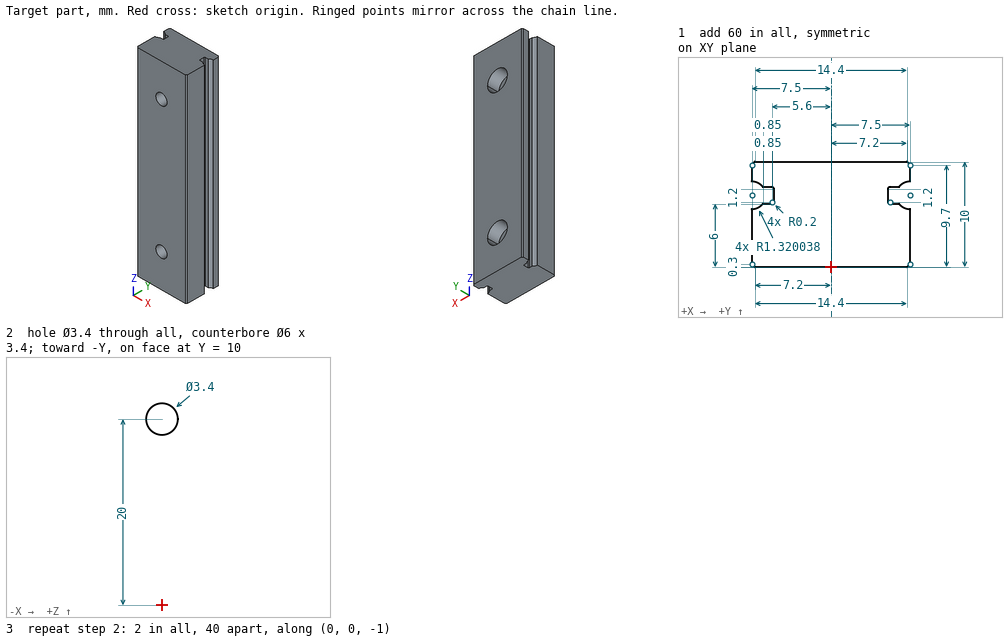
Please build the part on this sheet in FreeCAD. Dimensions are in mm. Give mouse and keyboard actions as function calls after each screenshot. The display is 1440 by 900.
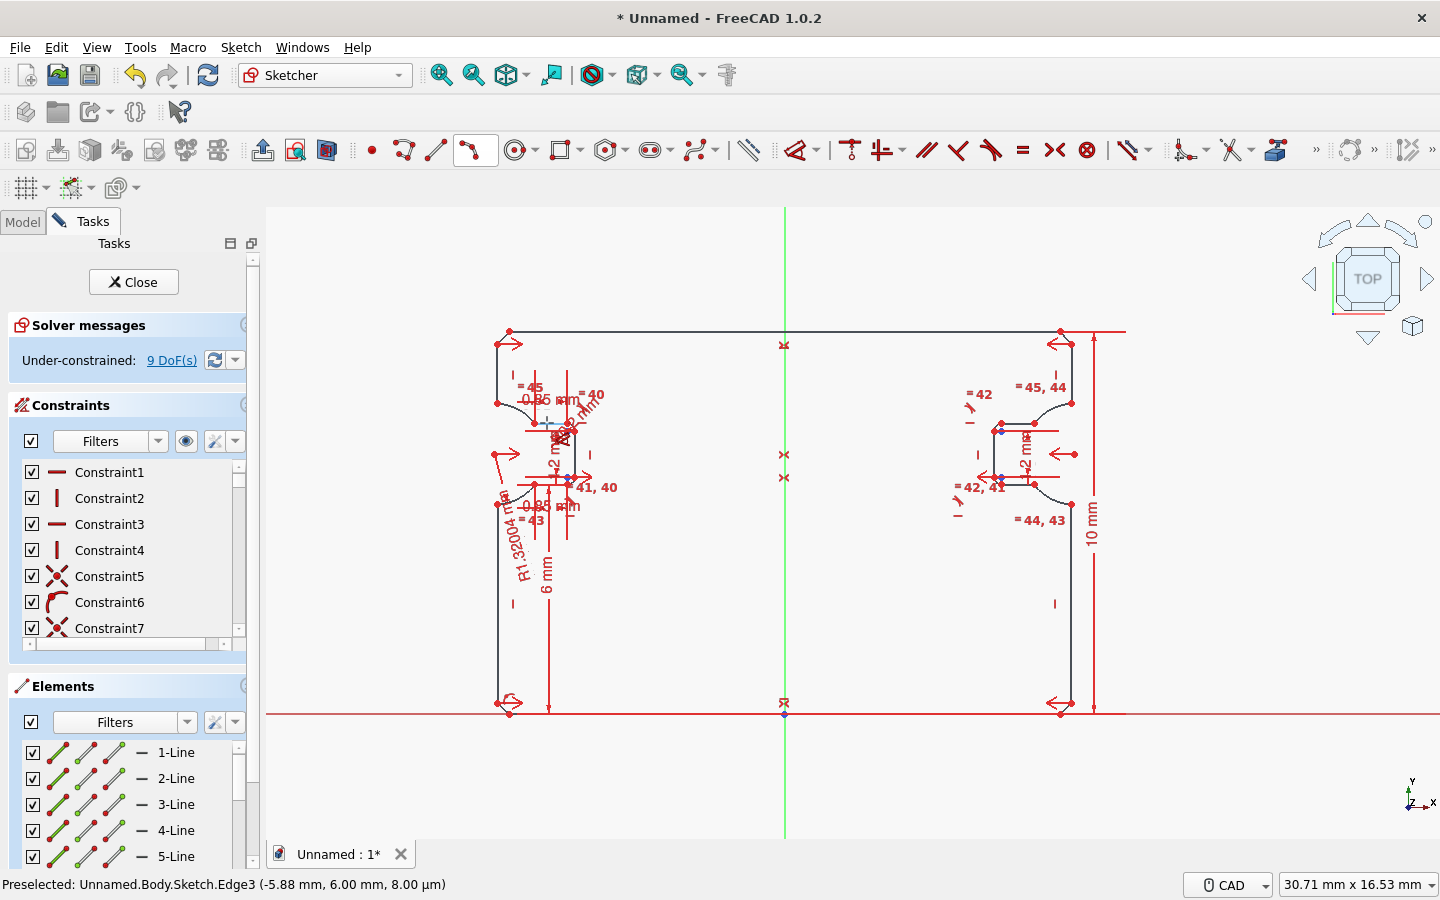
click(674, 714)
click(658, 748)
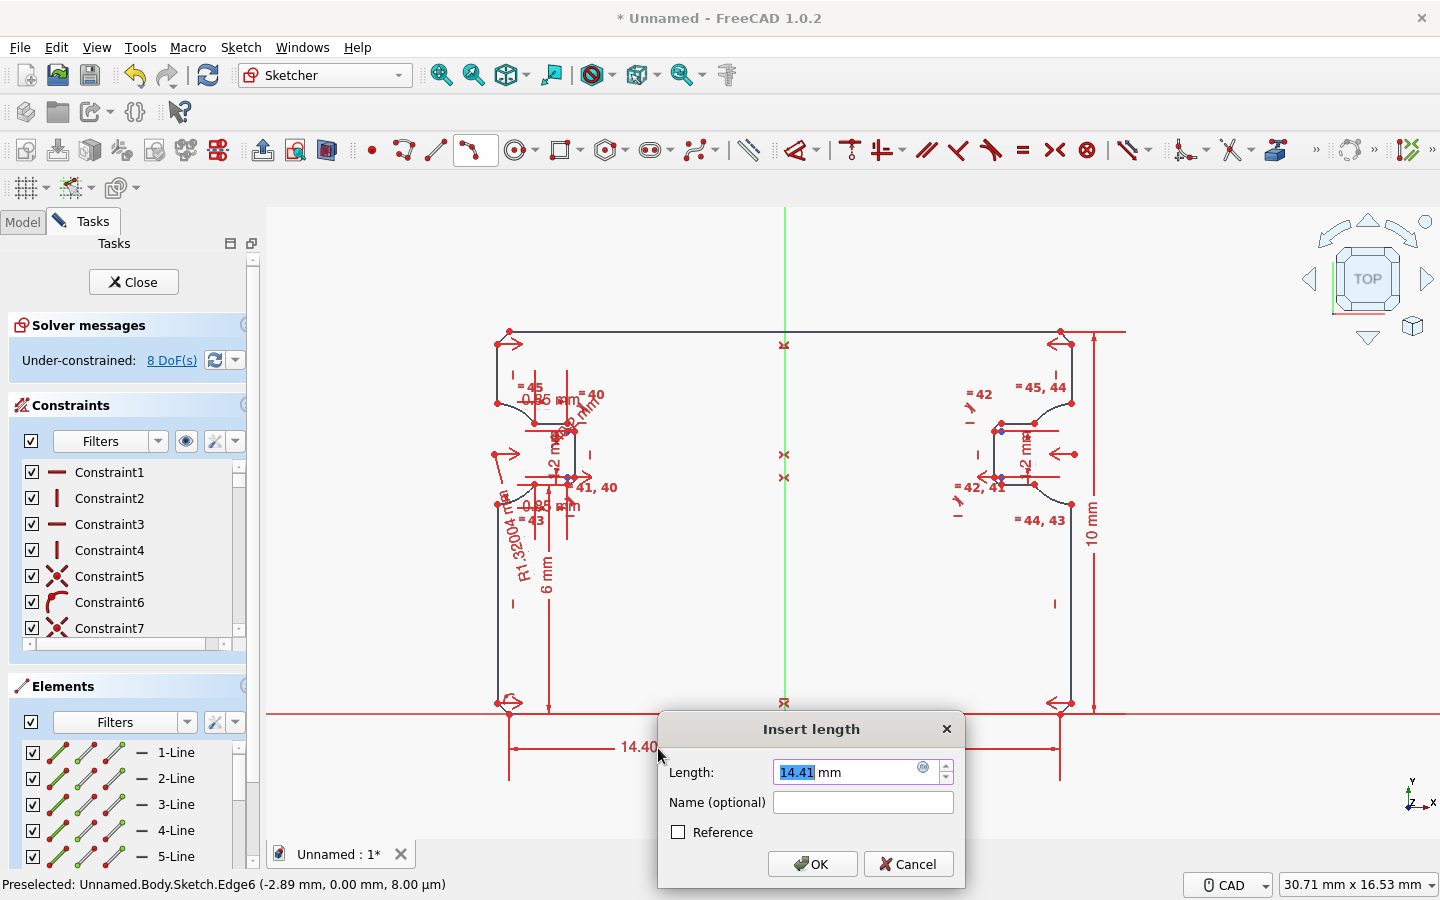
text(14.4)
key(Return)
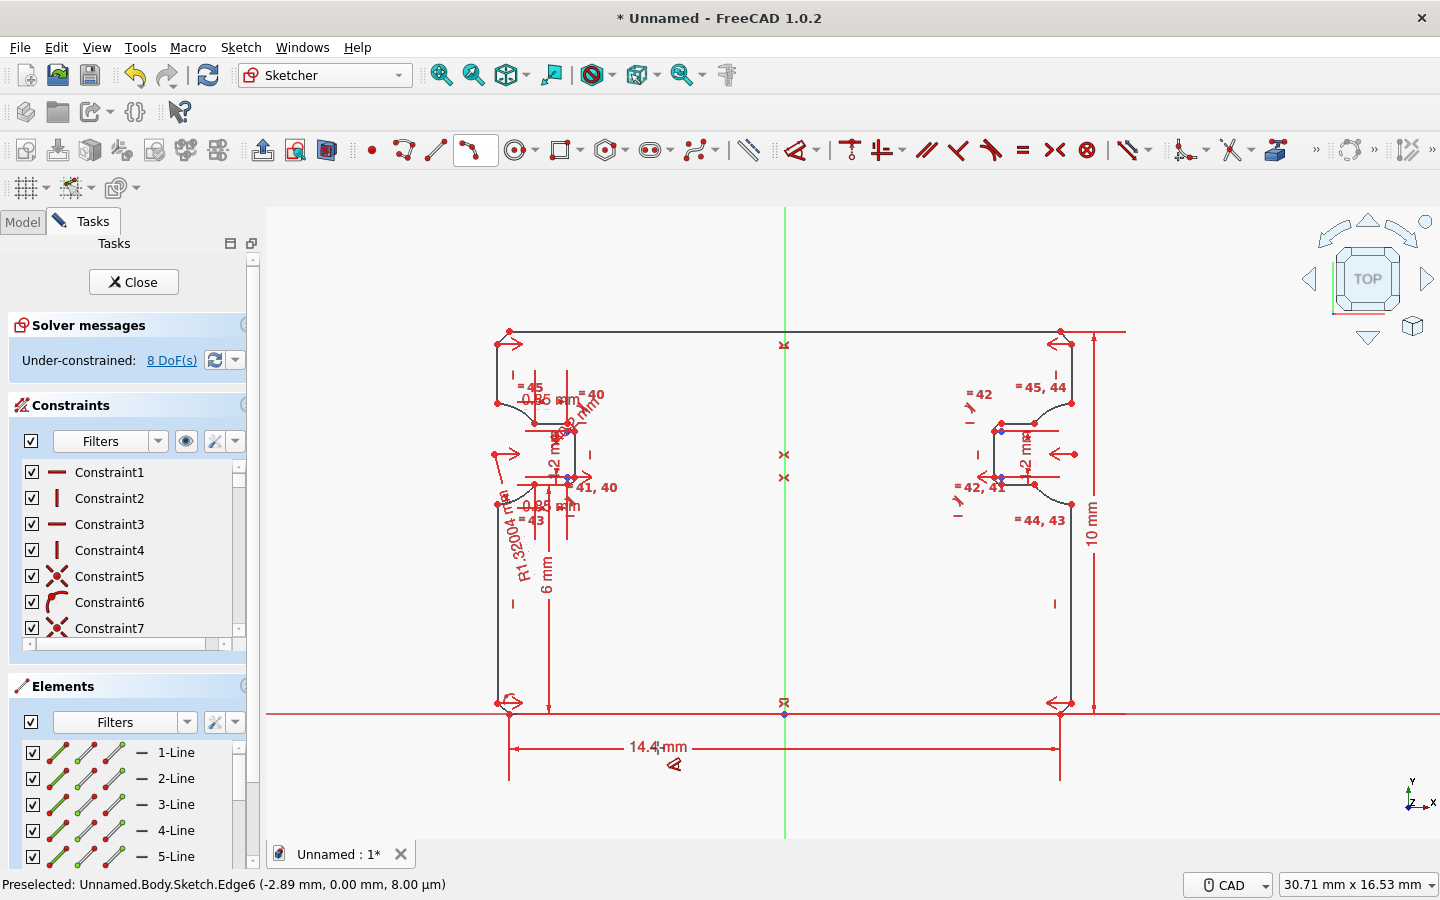
click(895, 332)
click(658, 298)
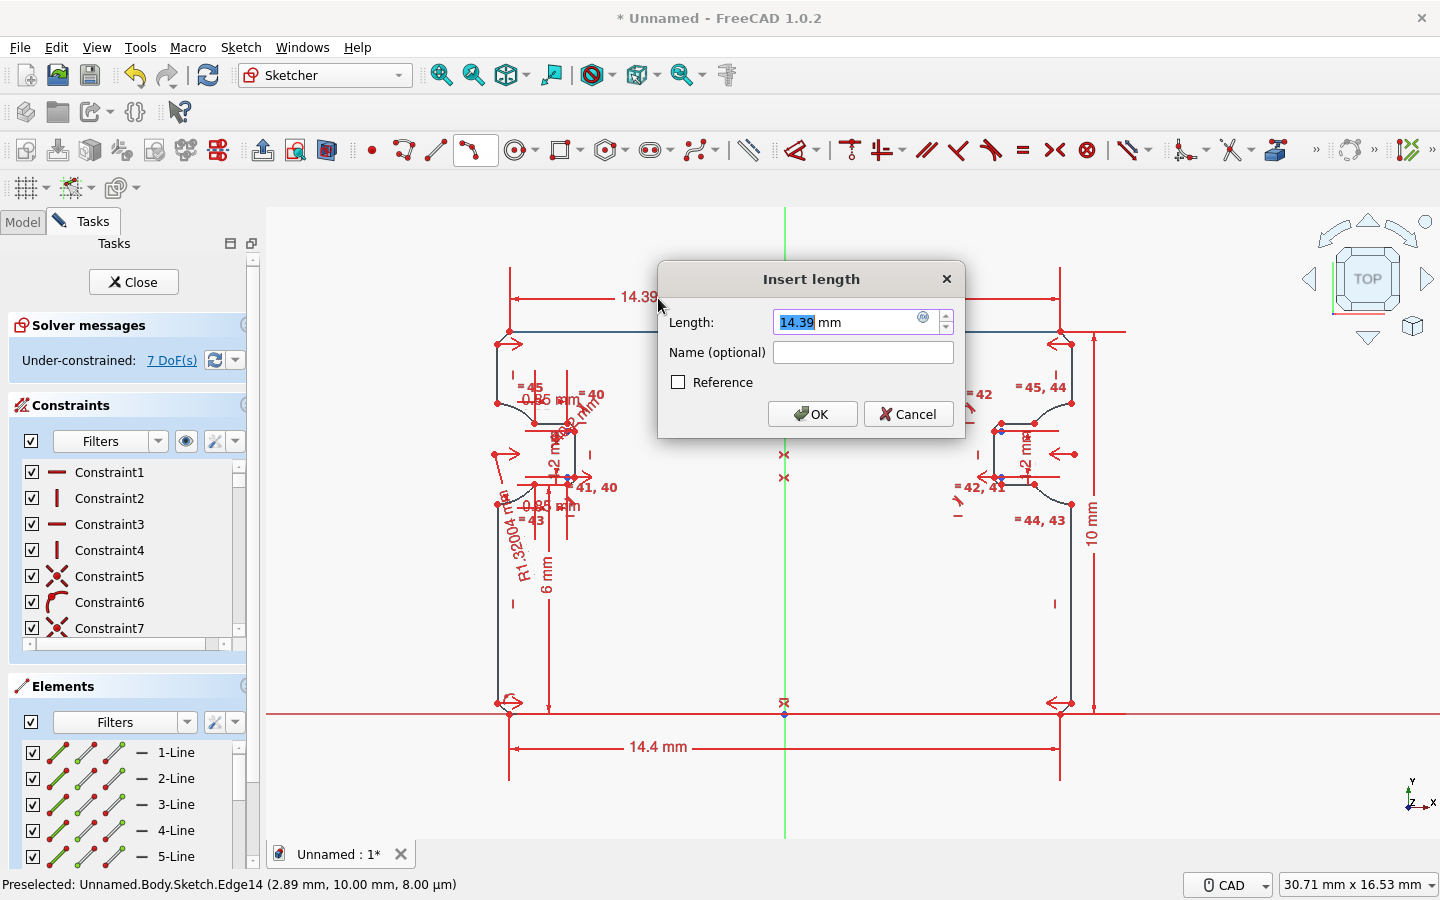
text(14.4)
key(Return)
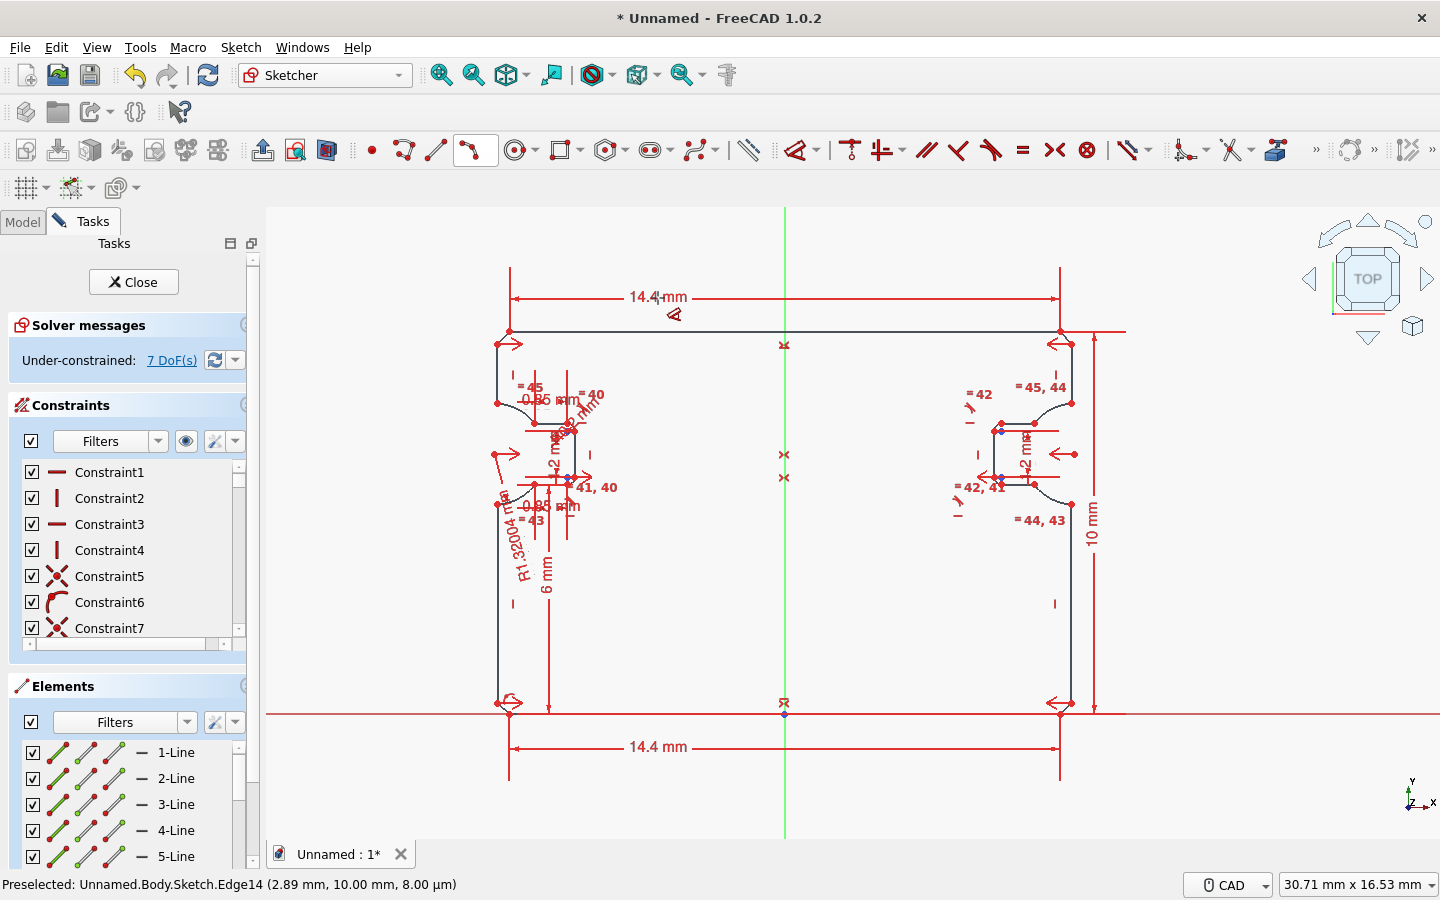
scroll(567, 424, up, 3)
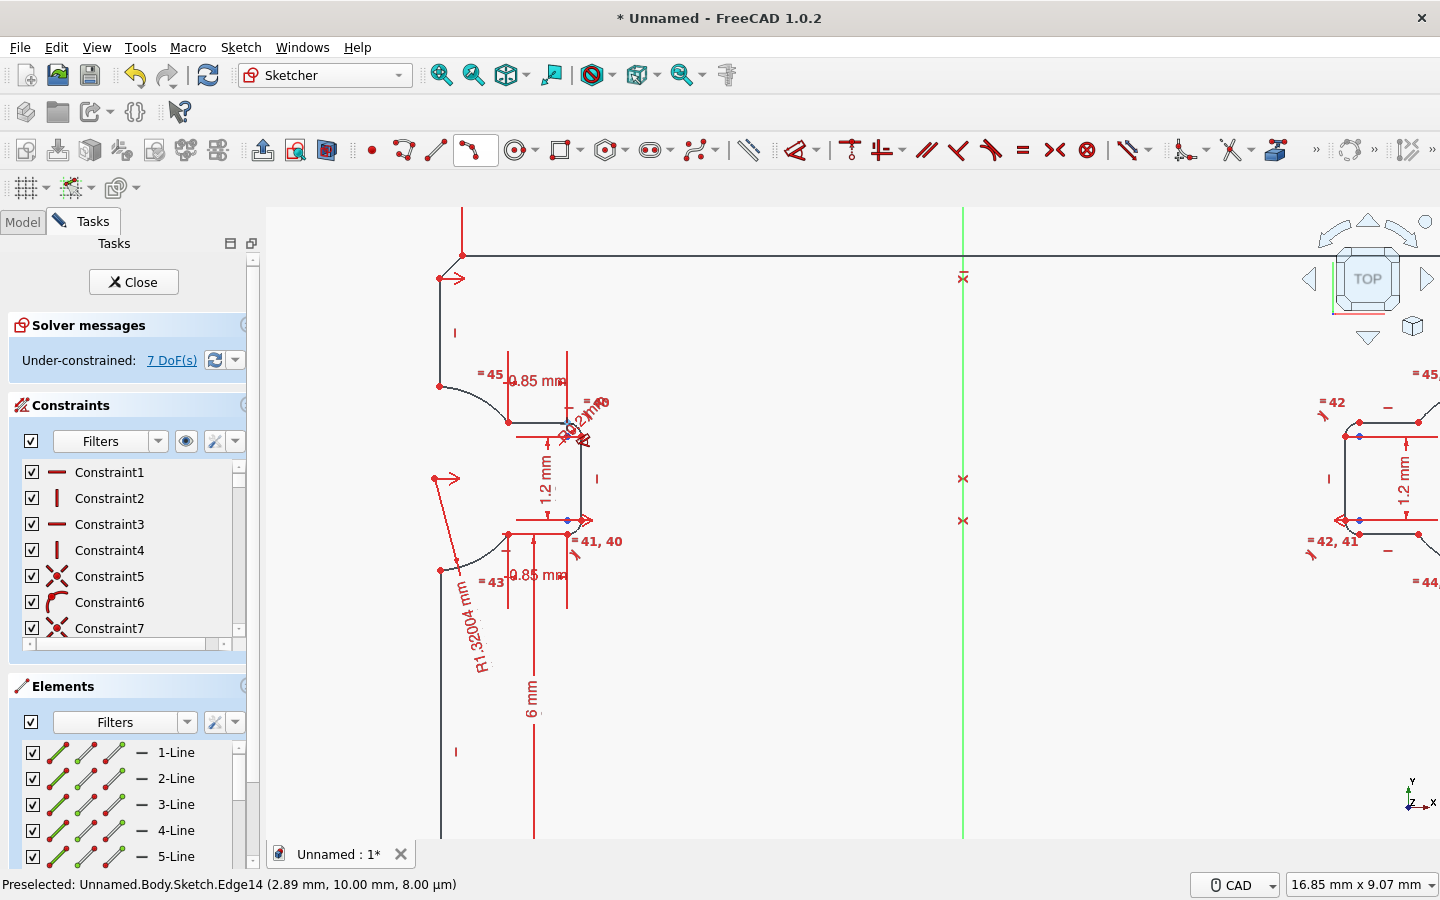
click(567, 423)
click(765, 389)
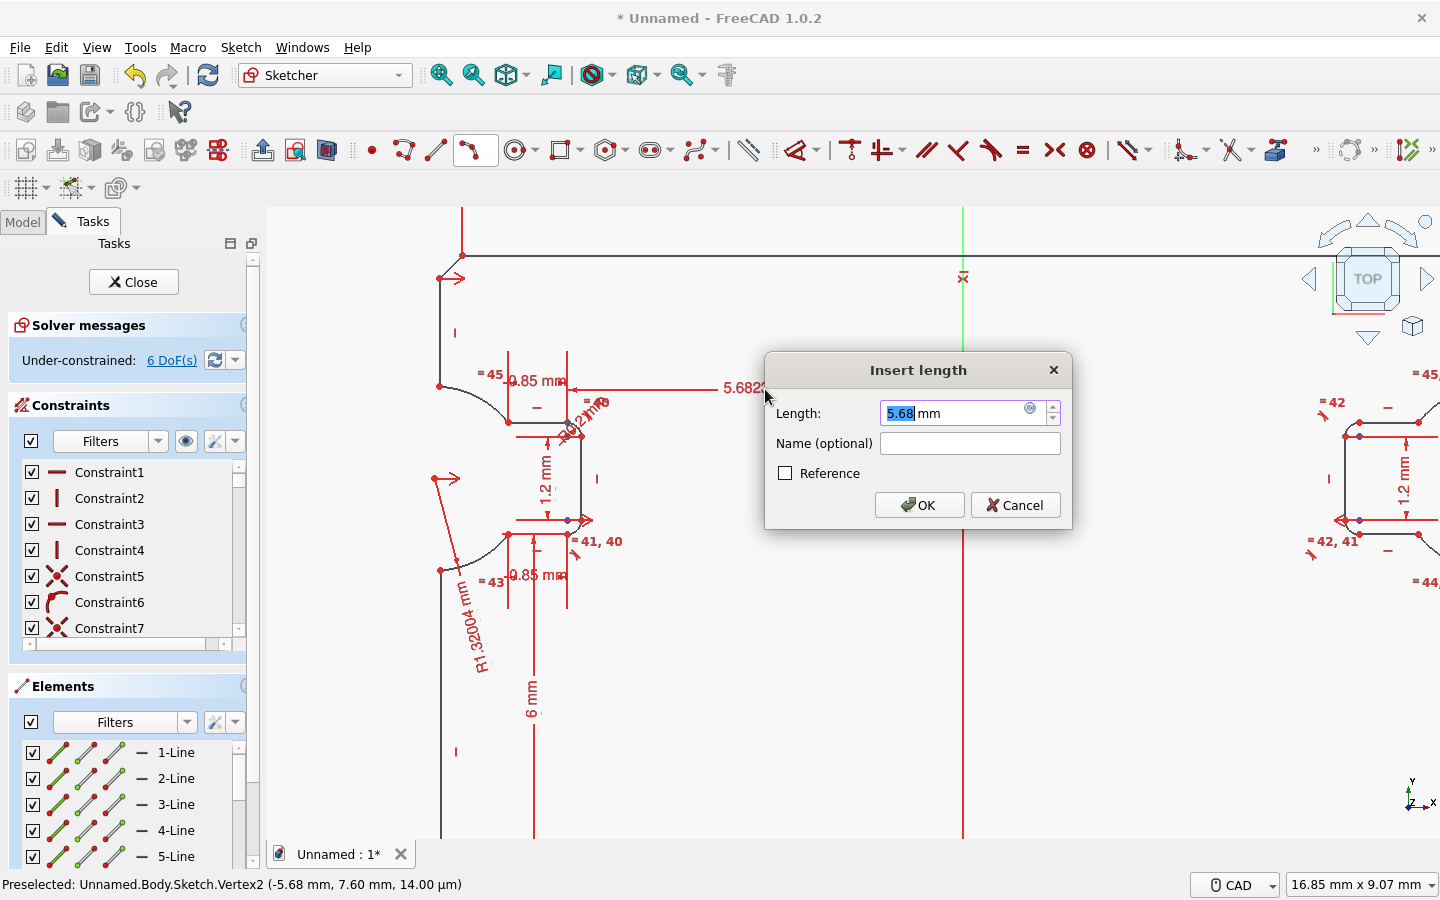
text(5.6)
key(Return)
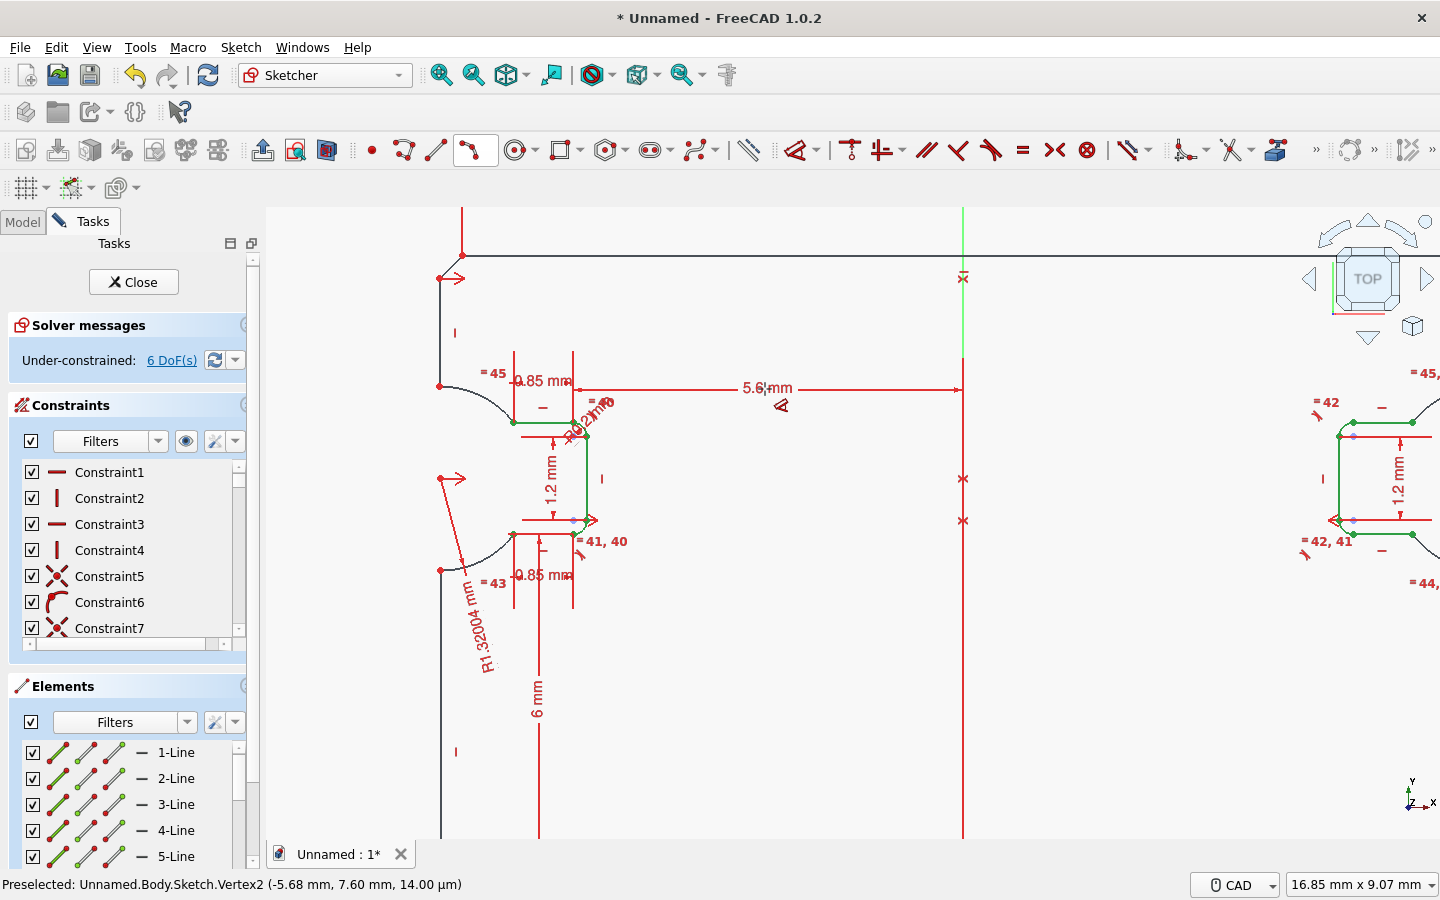
click(441, 571)
click(702, 537)